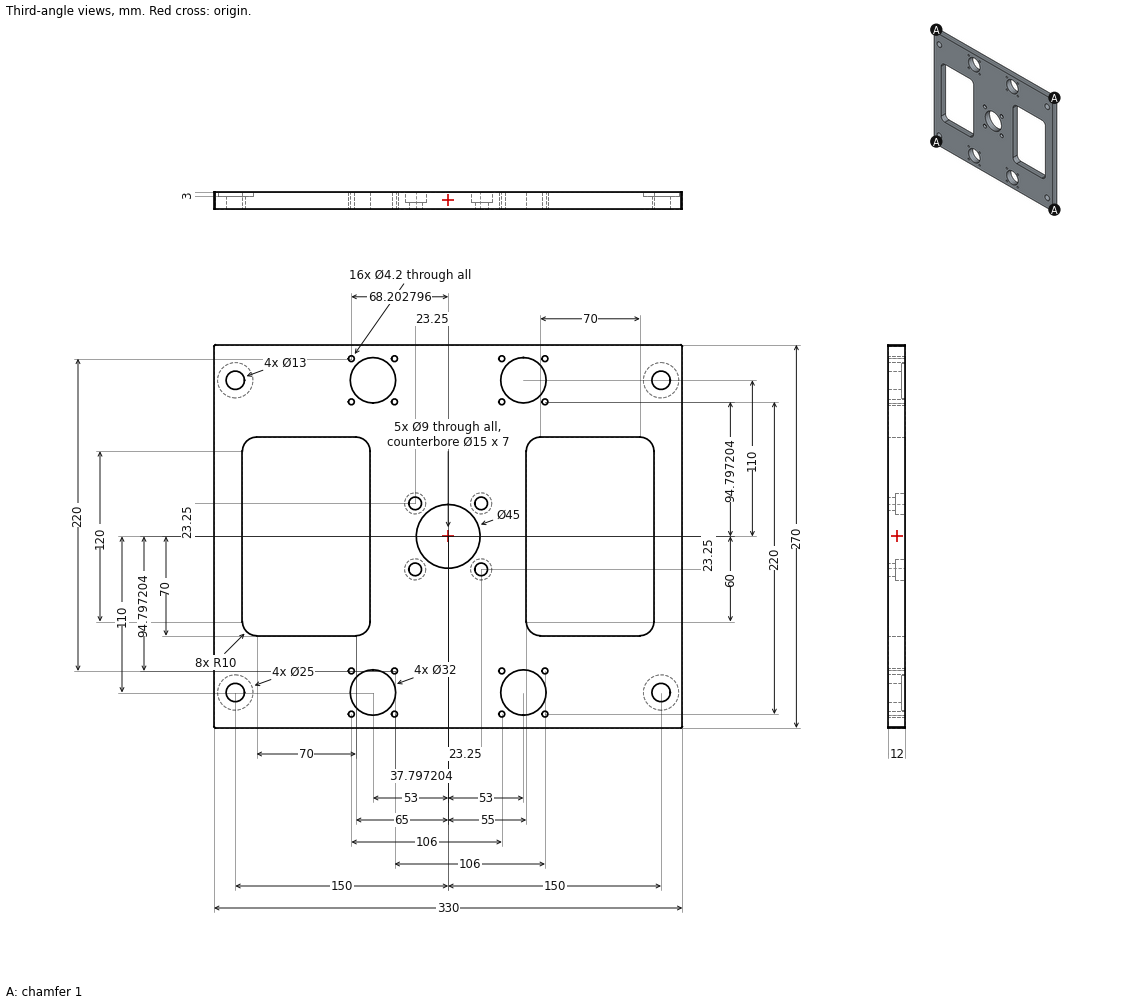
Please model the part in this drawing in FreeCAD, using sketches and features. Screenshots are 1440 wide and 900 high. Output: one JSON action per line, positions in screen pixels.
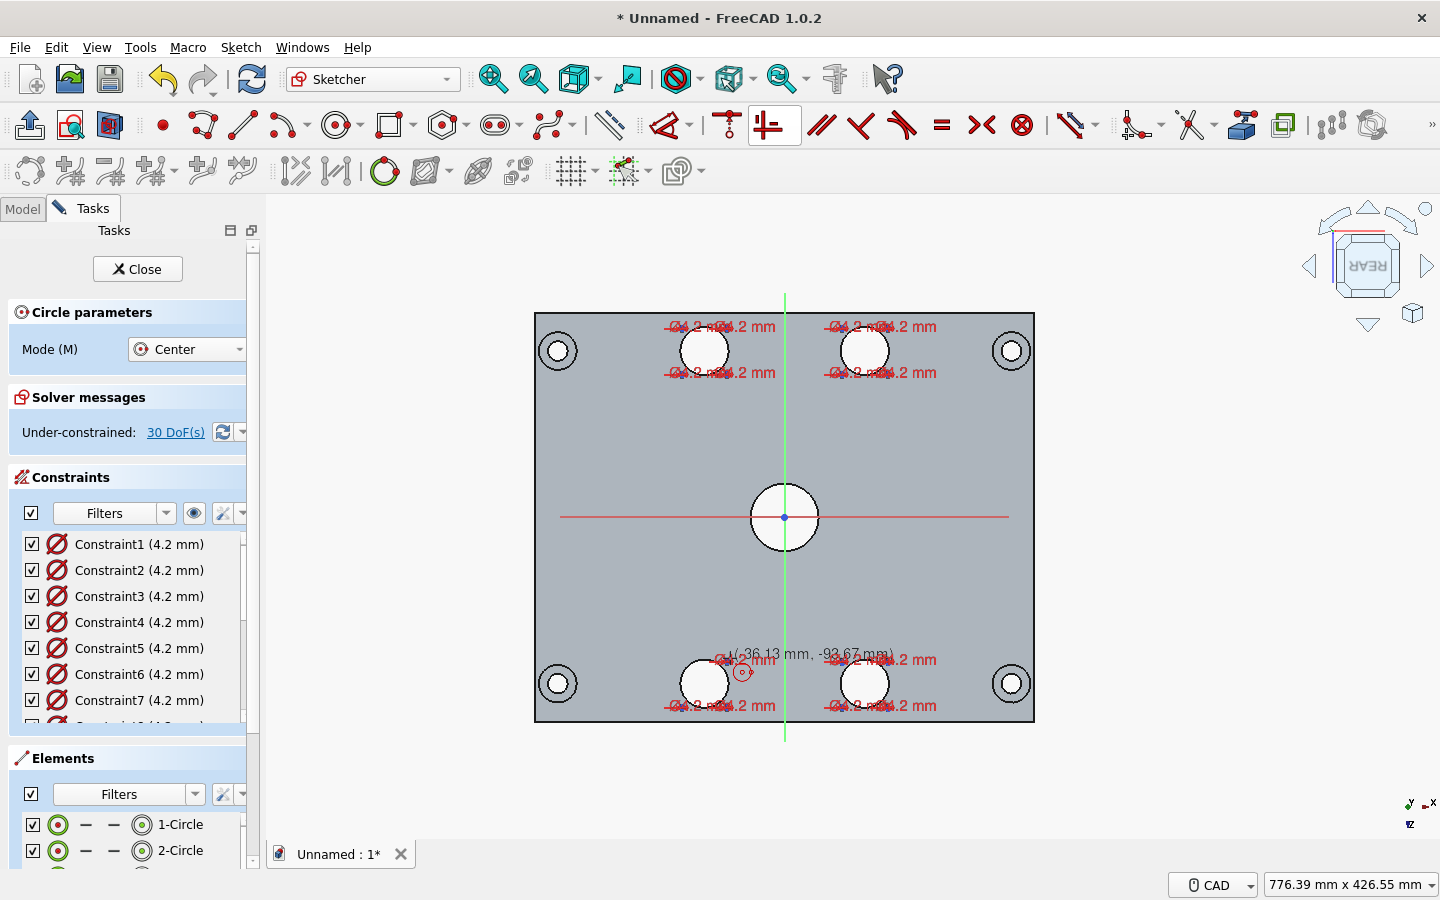
{"action": "scroll", "coordinate": [682, 661], "scroll_direction": "up", "scroll_amount": 10}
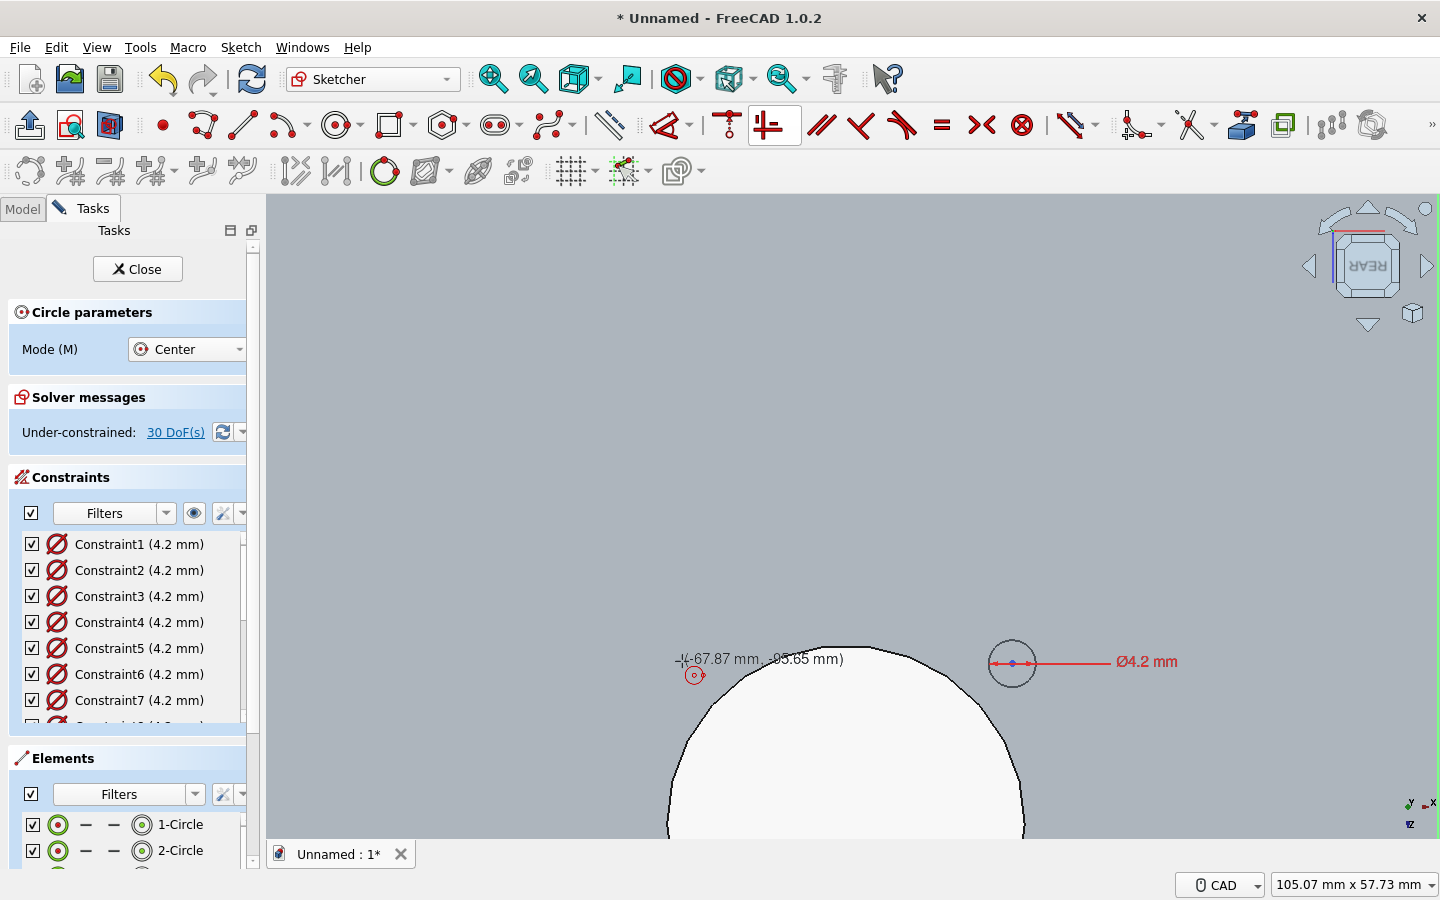
{"action": "scroll", "coordinate": [682, 661], "scroll_direction": "down", "scroll_amount": 10}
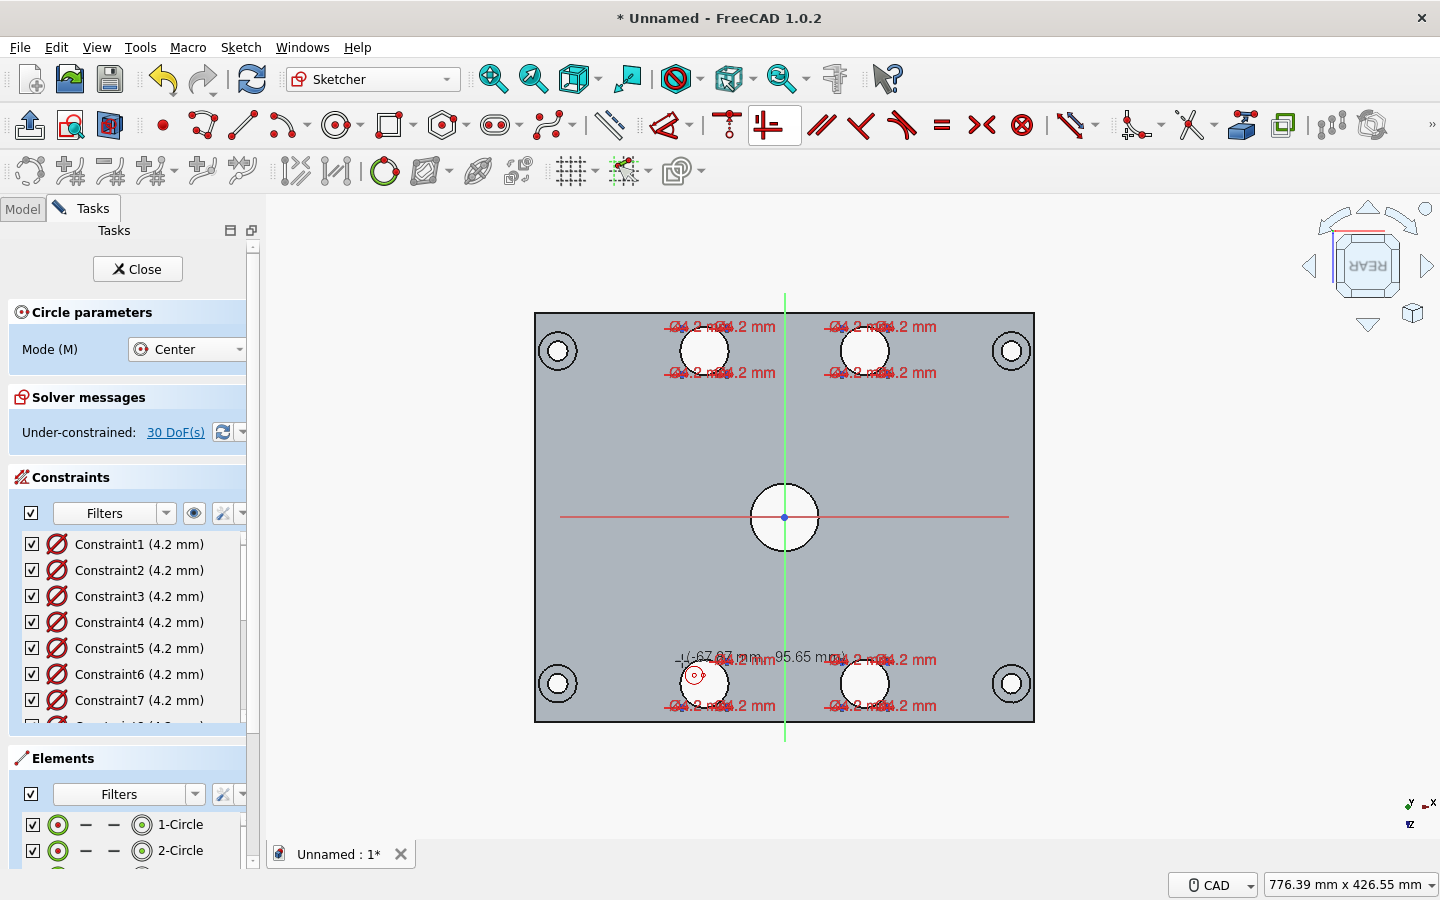
{"action": "left_click", "coordinate": [682, 661]}
{"action": "mouse_move", "coordinate": [684, 658]}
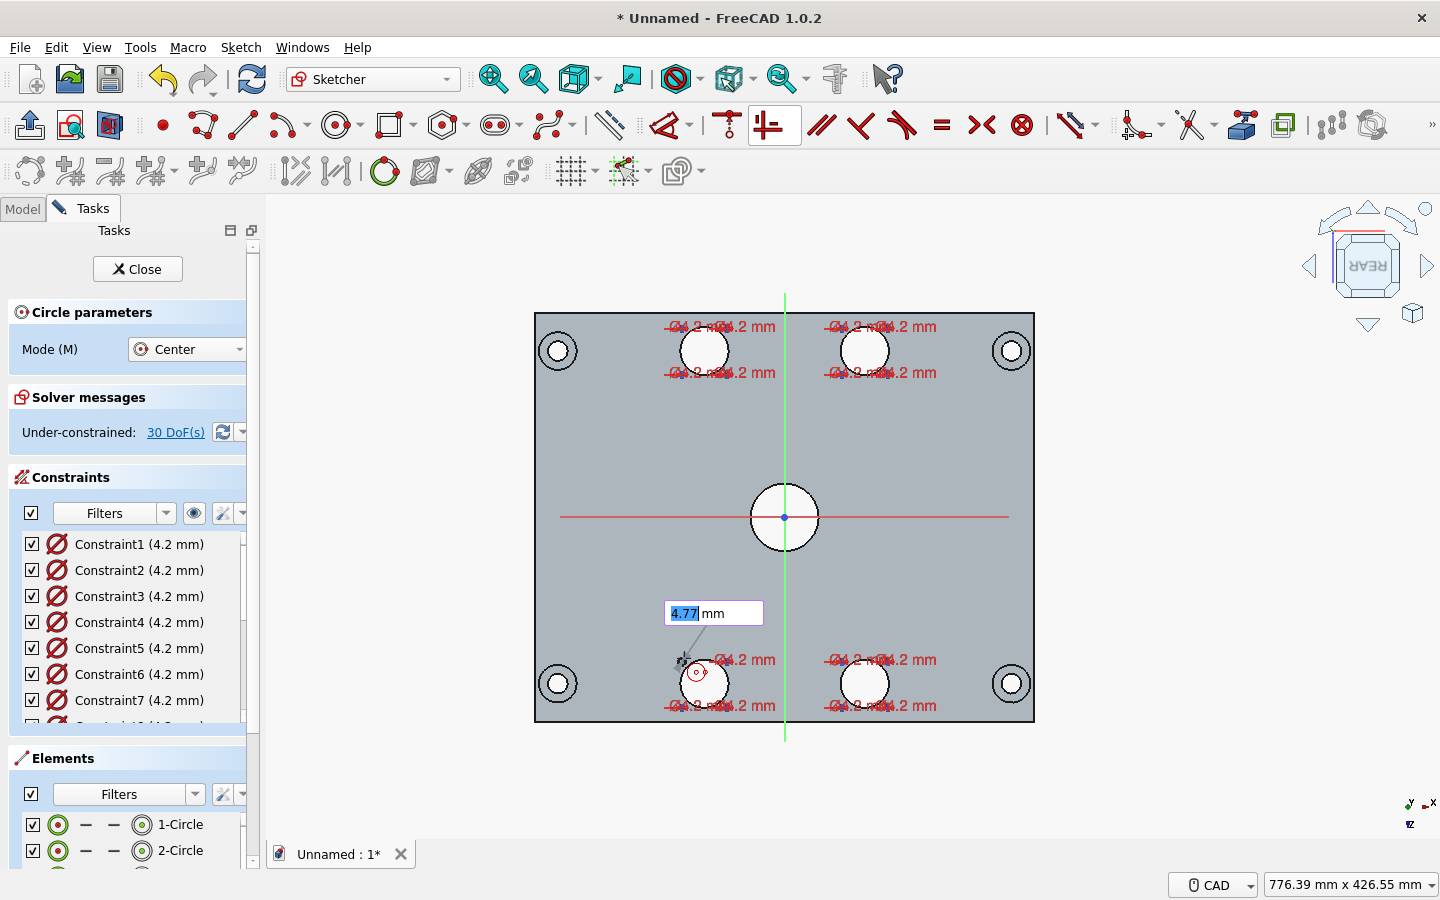
{"action": "type", "text": "4.2"}
{"action": "key", "text": "Return"}
{"action": "key", "text": "Escape"}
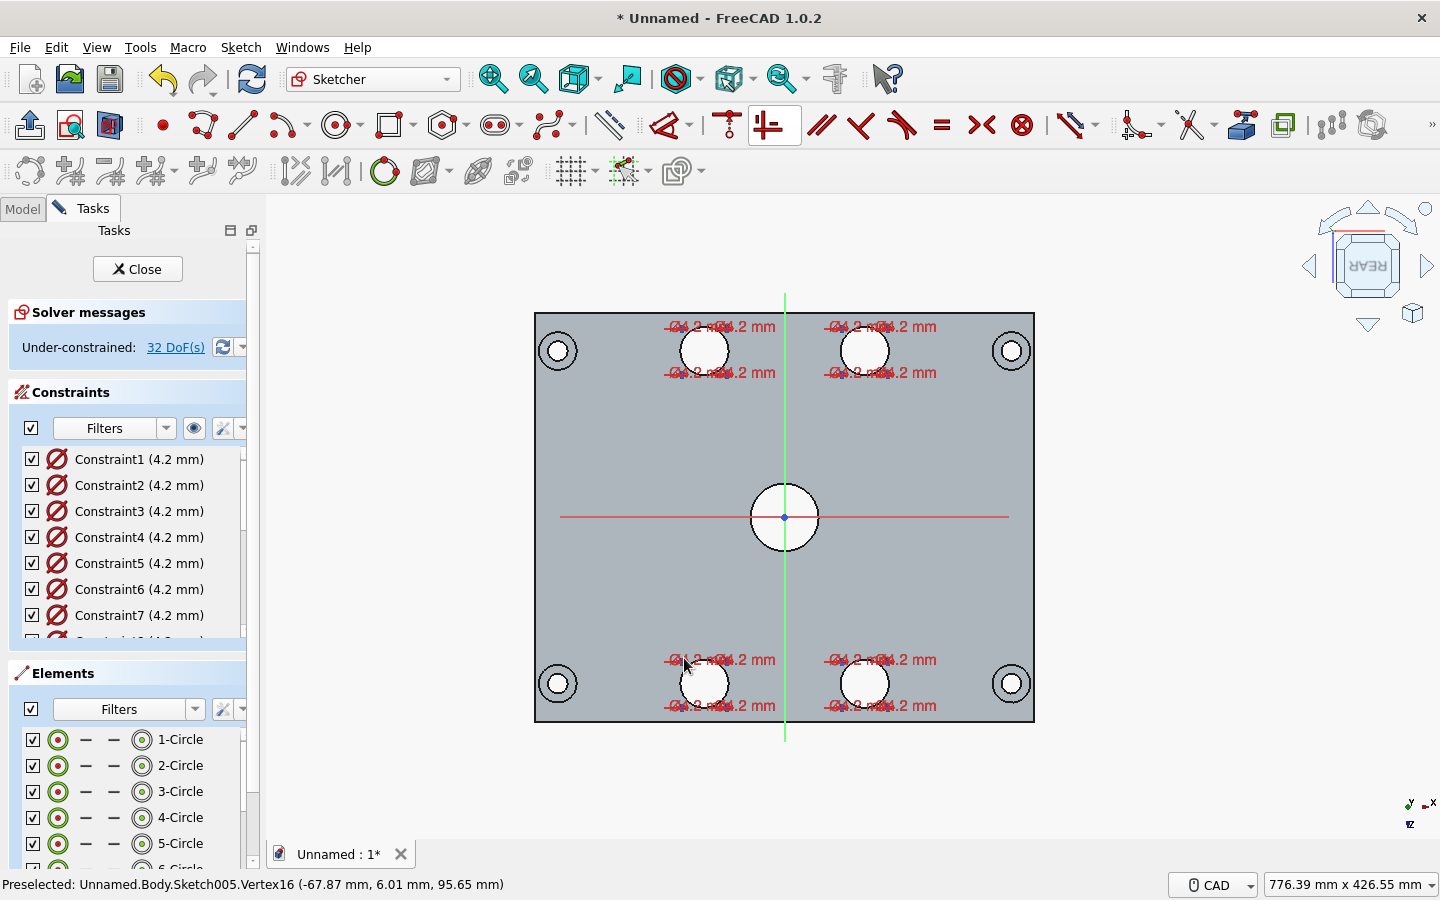
{"action": "left_click", "coordinate": [682, 708]}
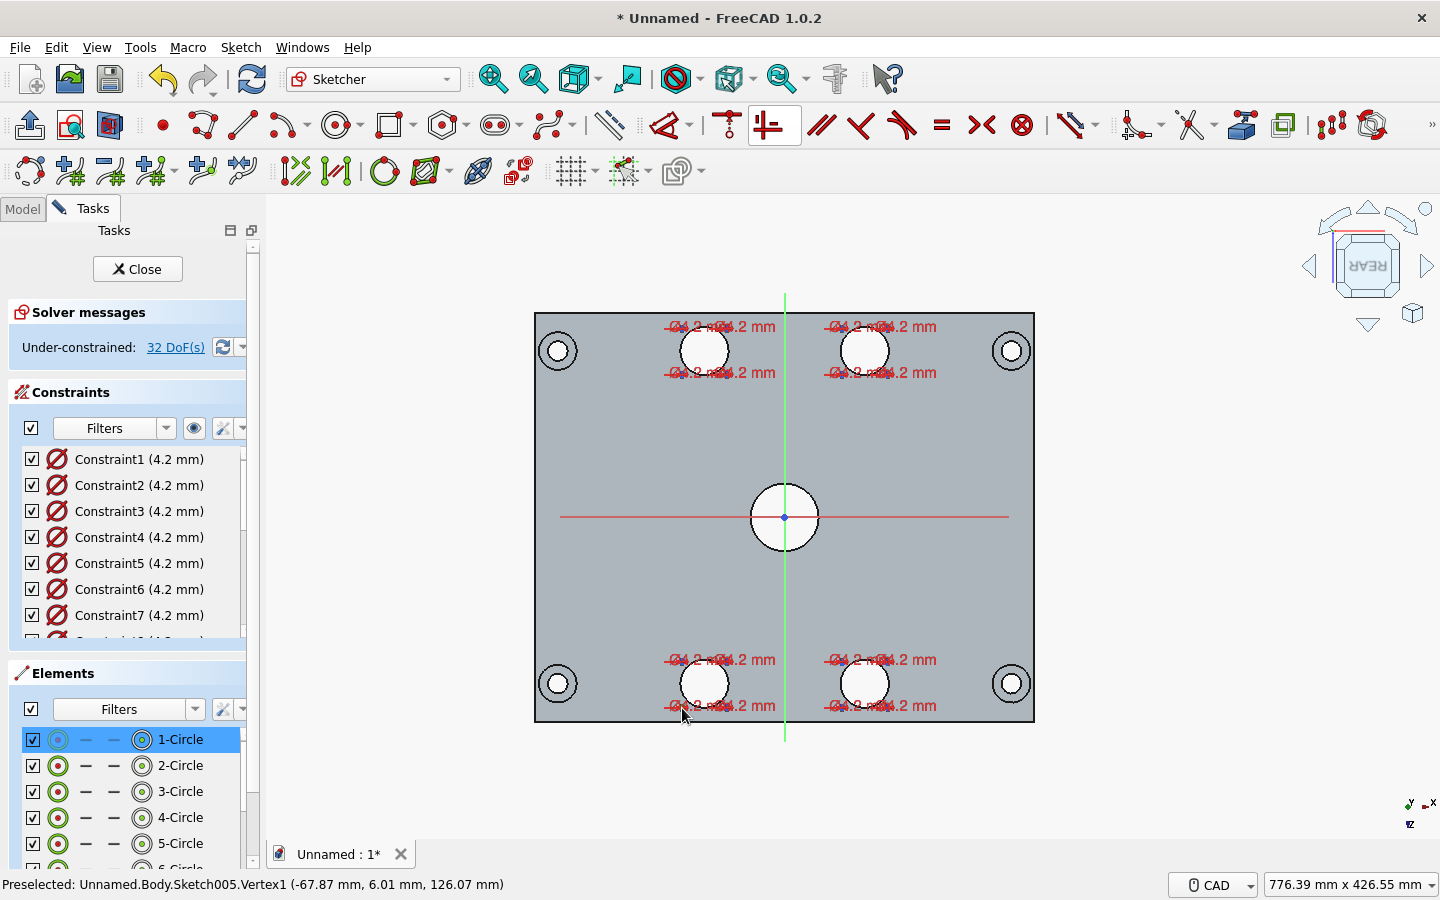
{"action": "left_click", "coordinate": [682, 329]}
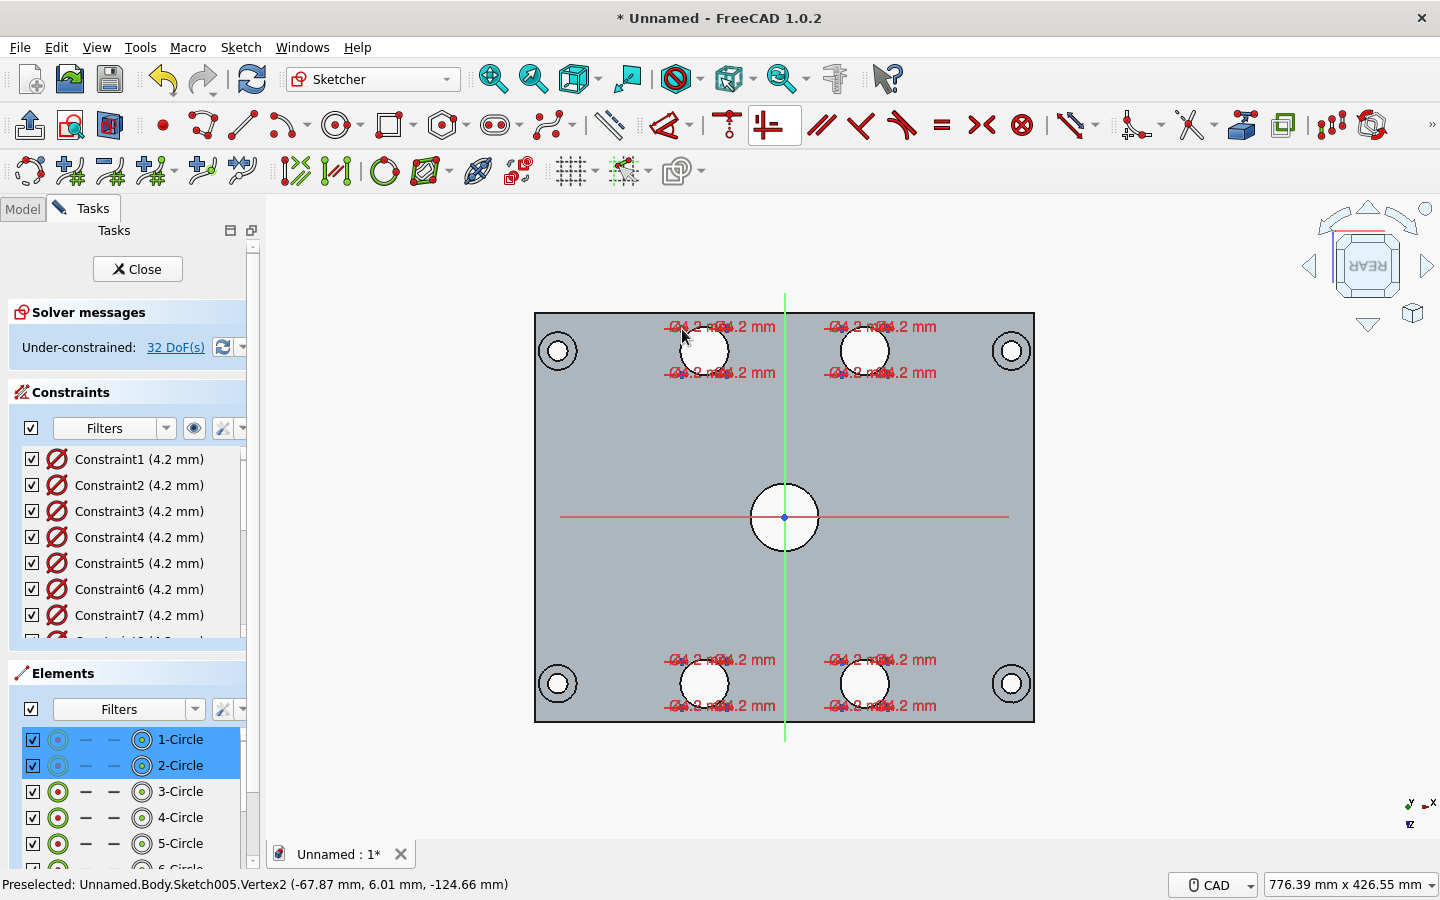
{"action": "key", "text": "v"}